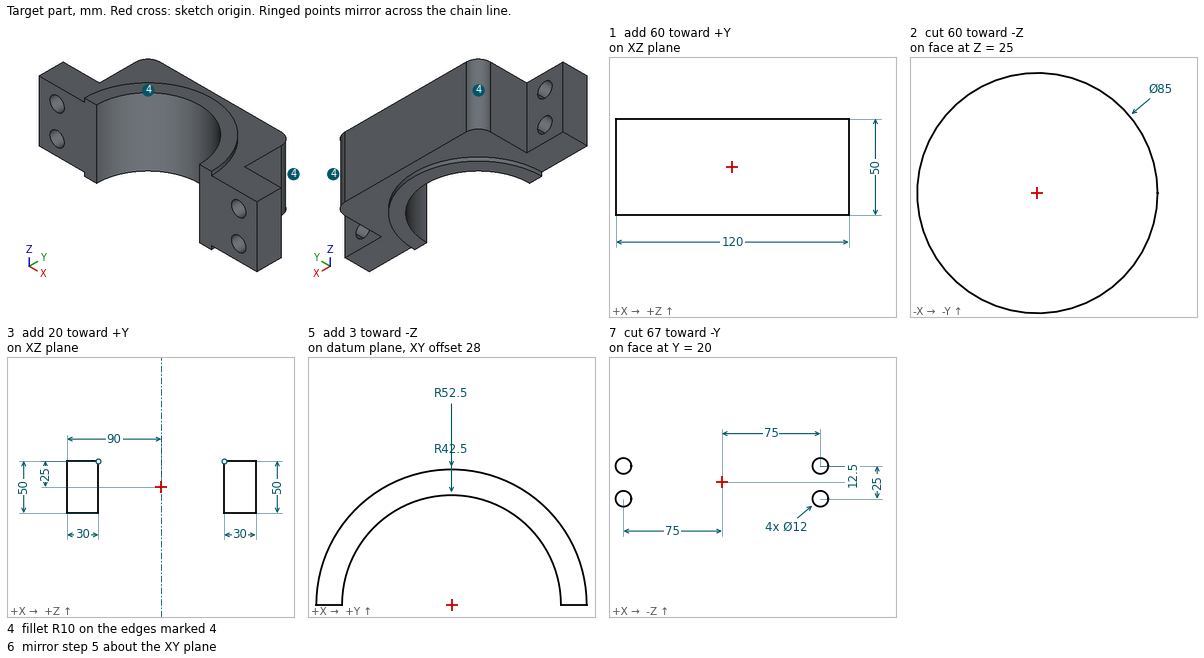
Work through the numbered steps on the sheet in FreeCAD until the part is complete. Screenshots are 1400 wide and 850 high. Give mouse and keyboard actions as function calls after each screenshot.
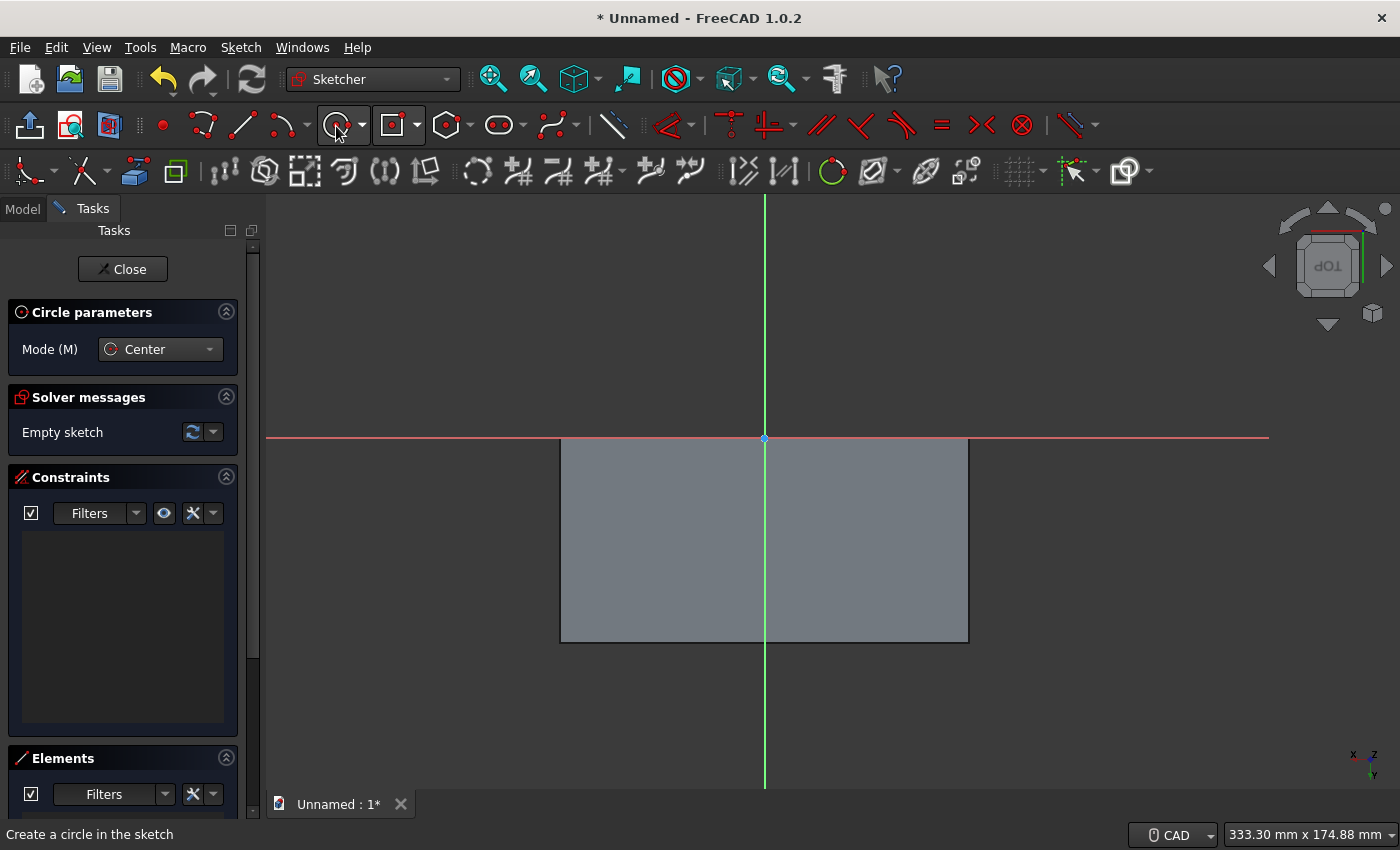
click(765, 438)
move(867, 336)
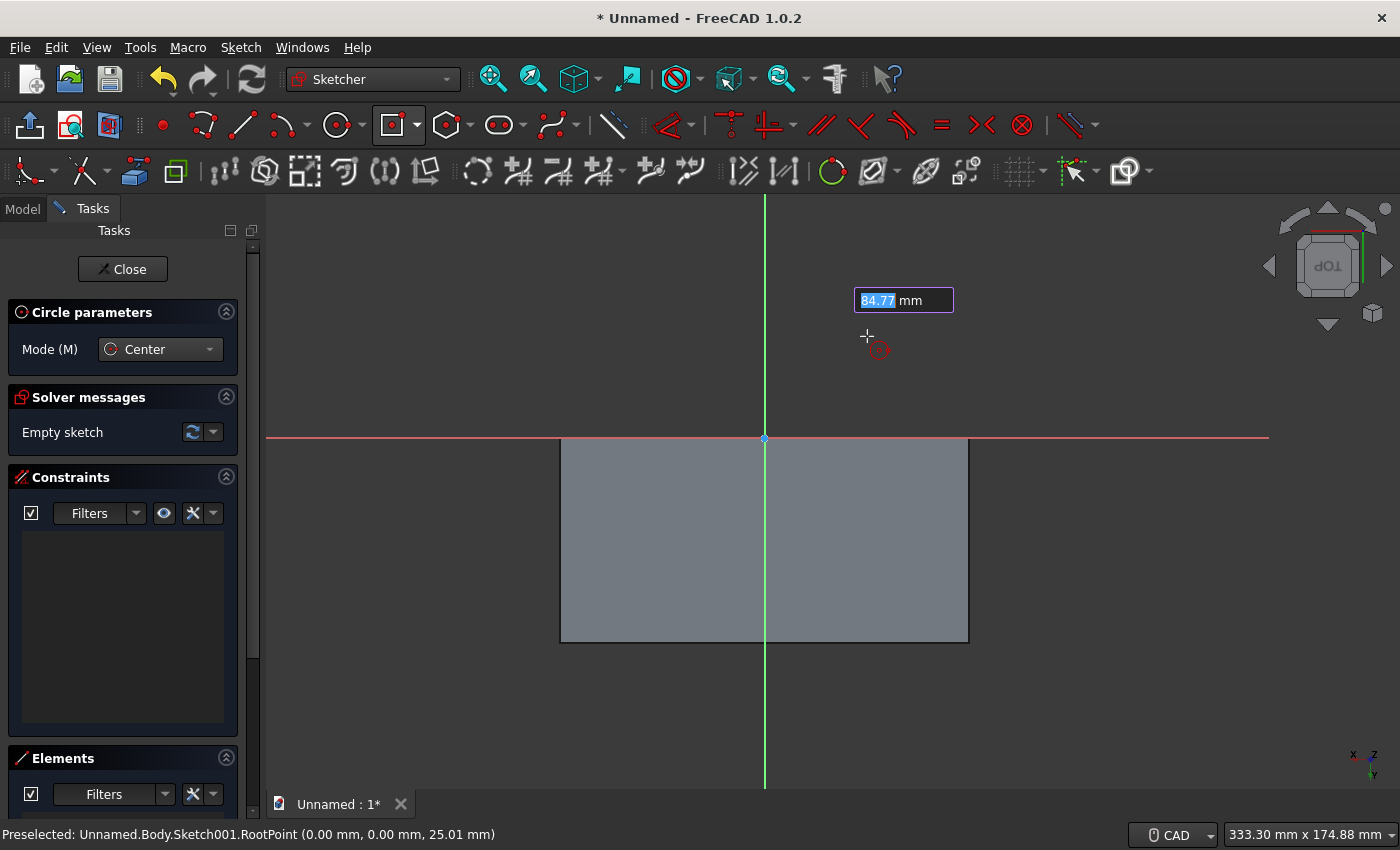
text(85)
key(Return)
key(Escape)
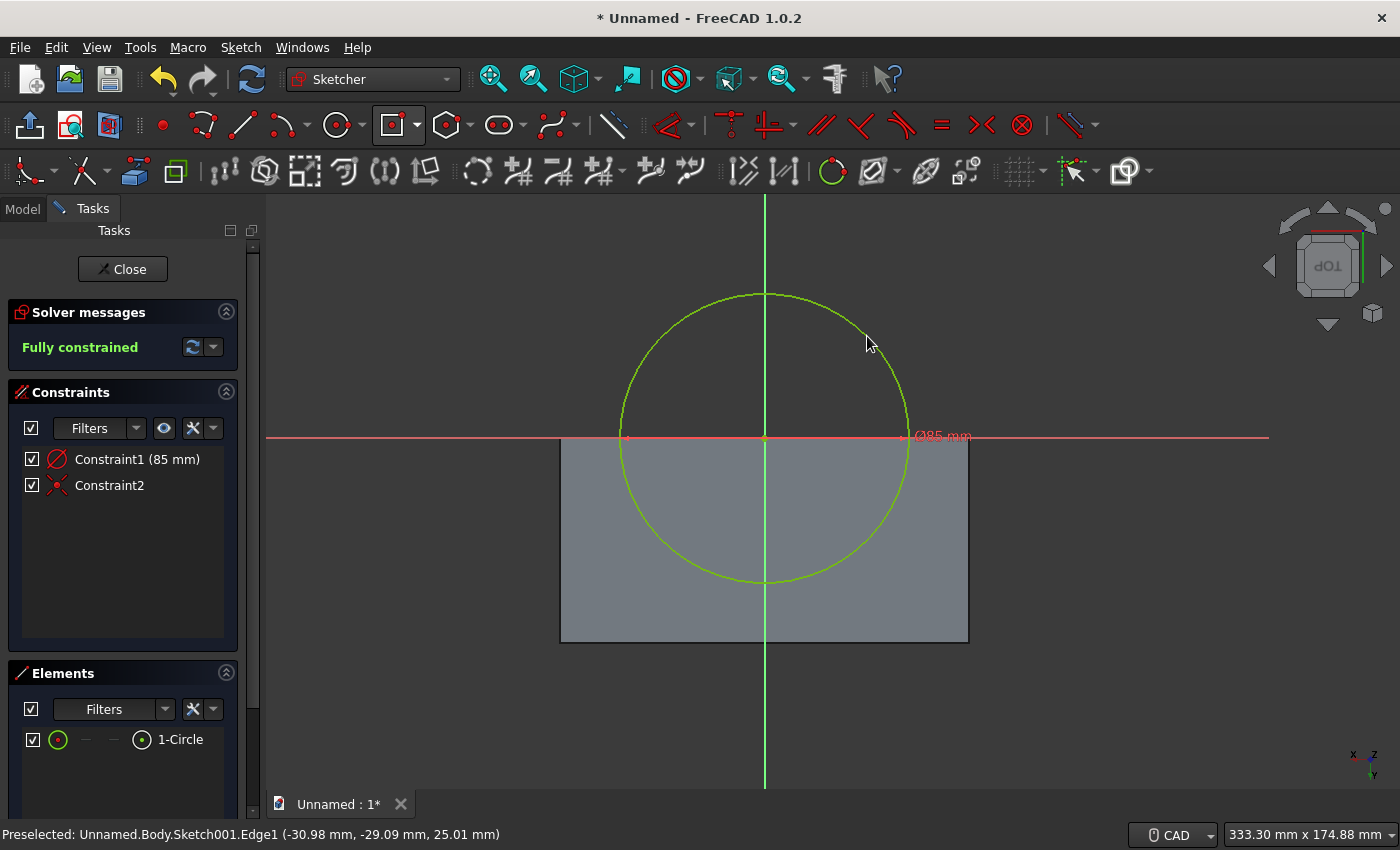
click(123, 269)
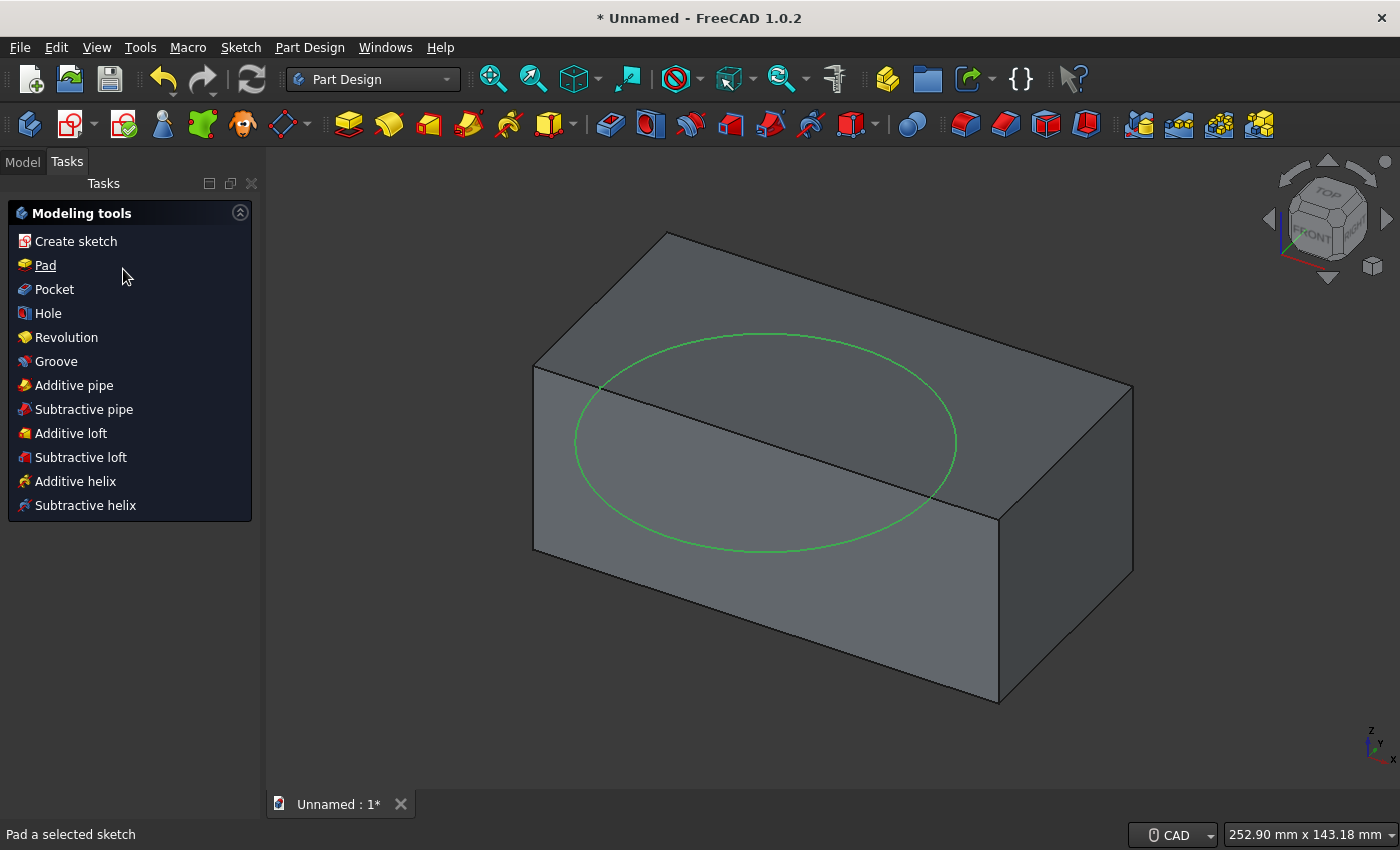
click(612, 124)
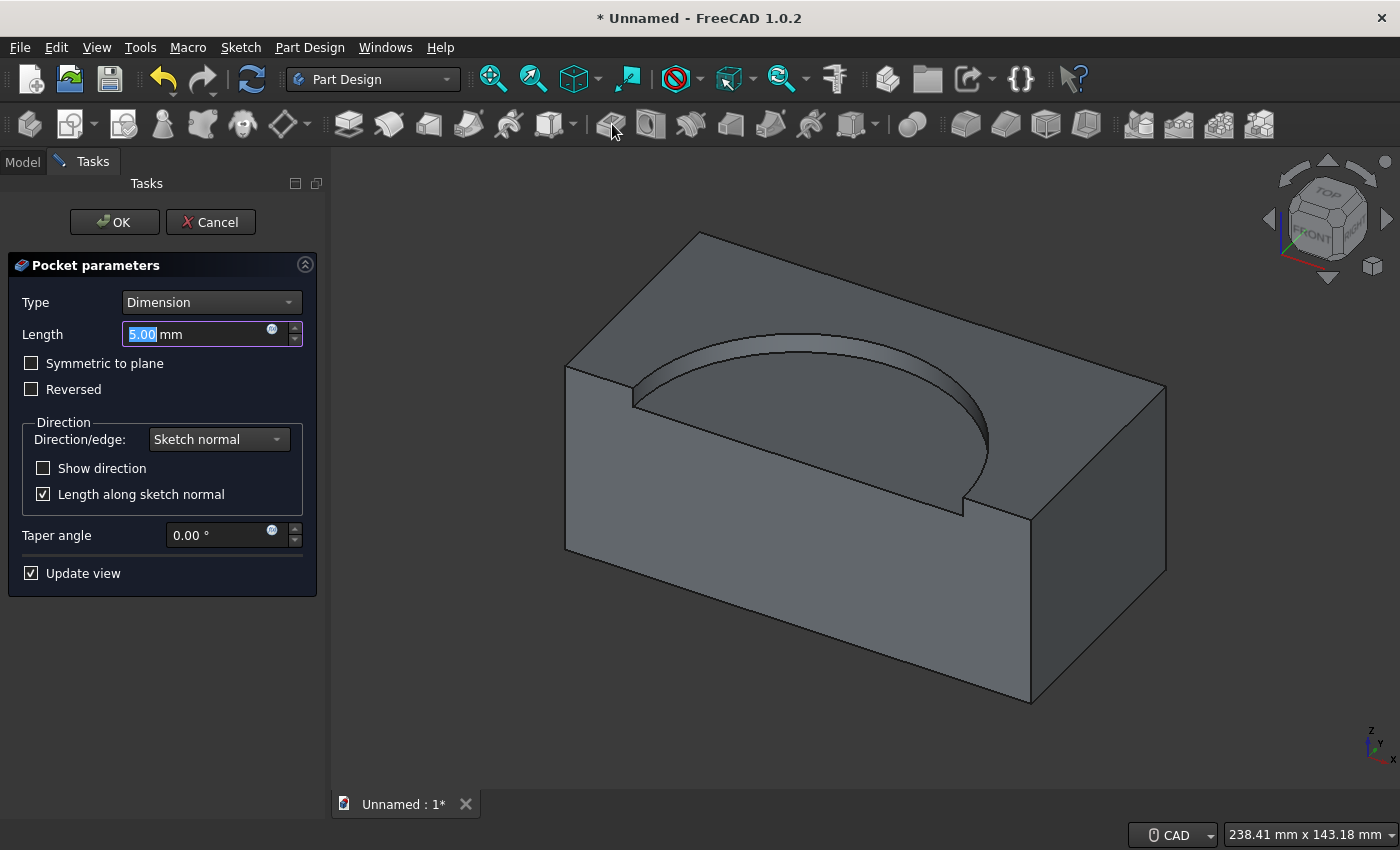
text(60)
key(Tab)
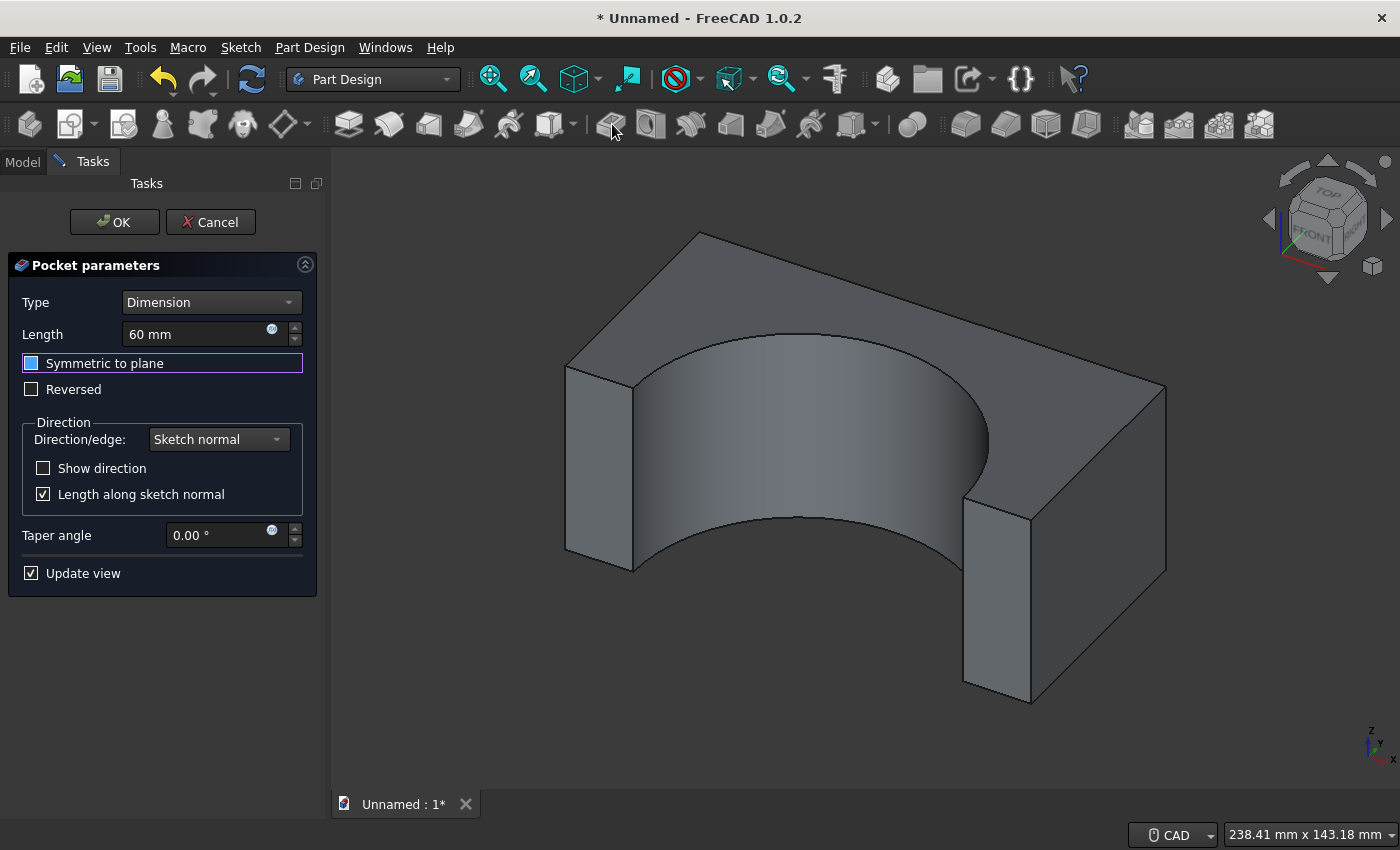
click(115, 222)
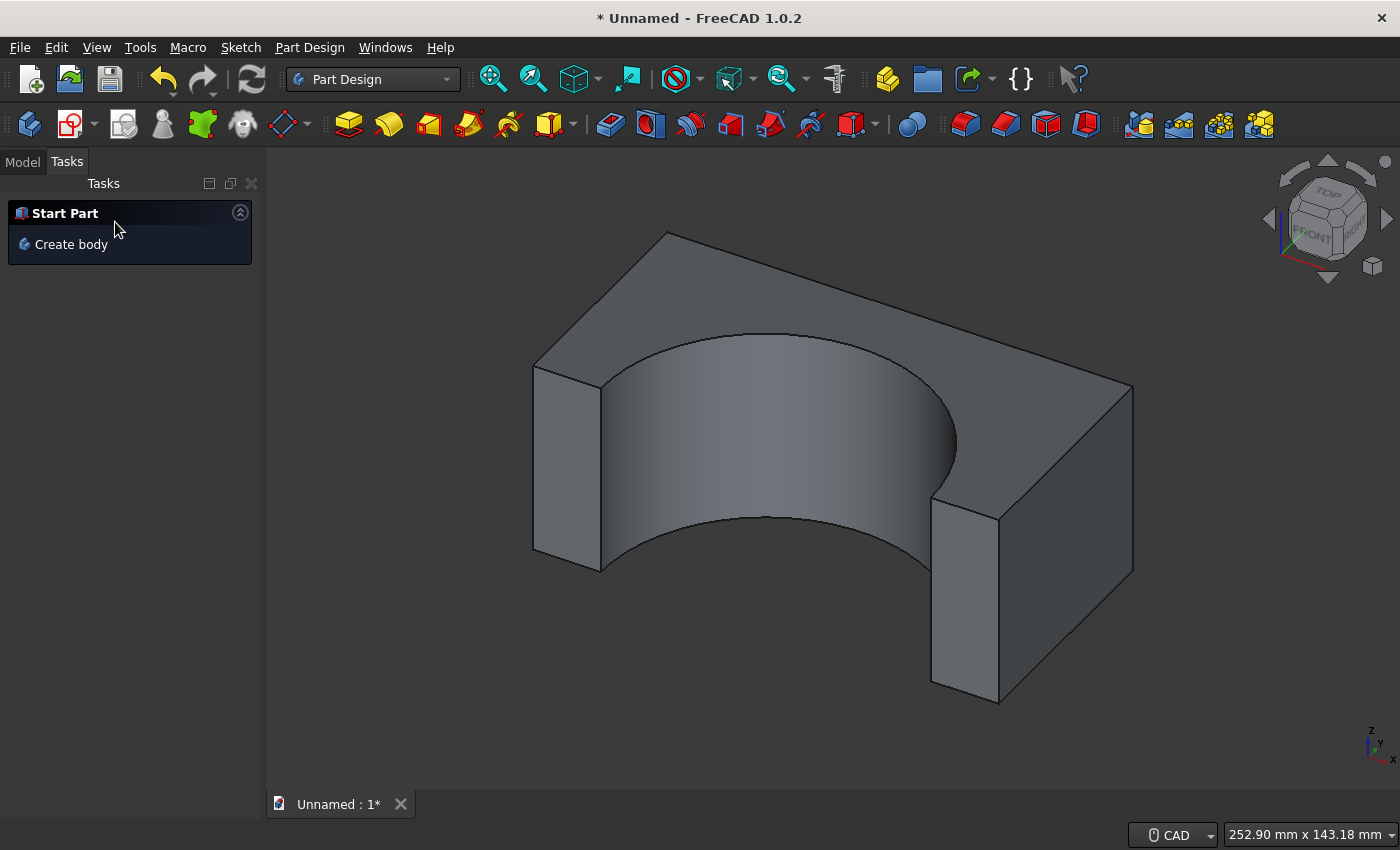
click(70, 124)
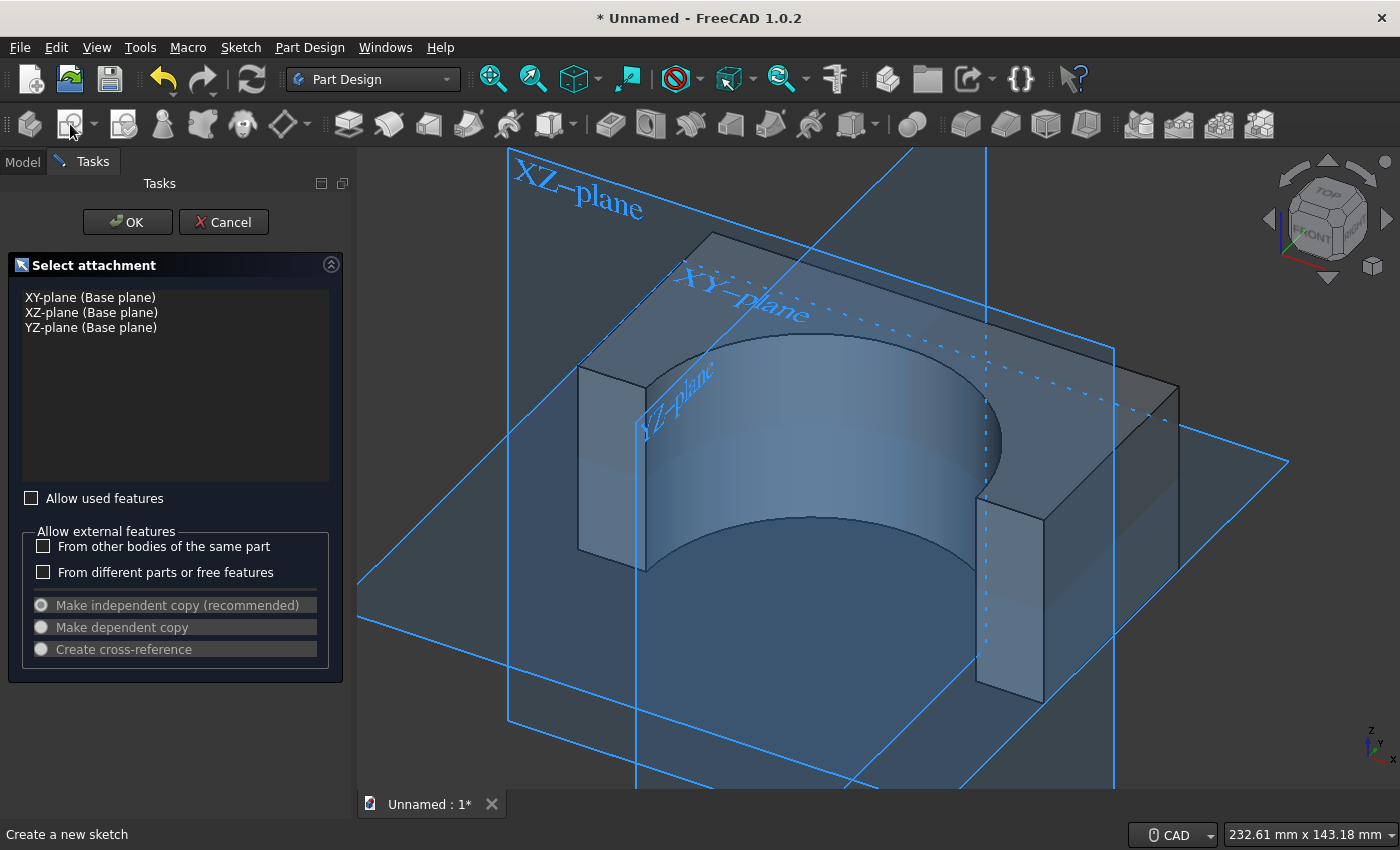
click(82, 312)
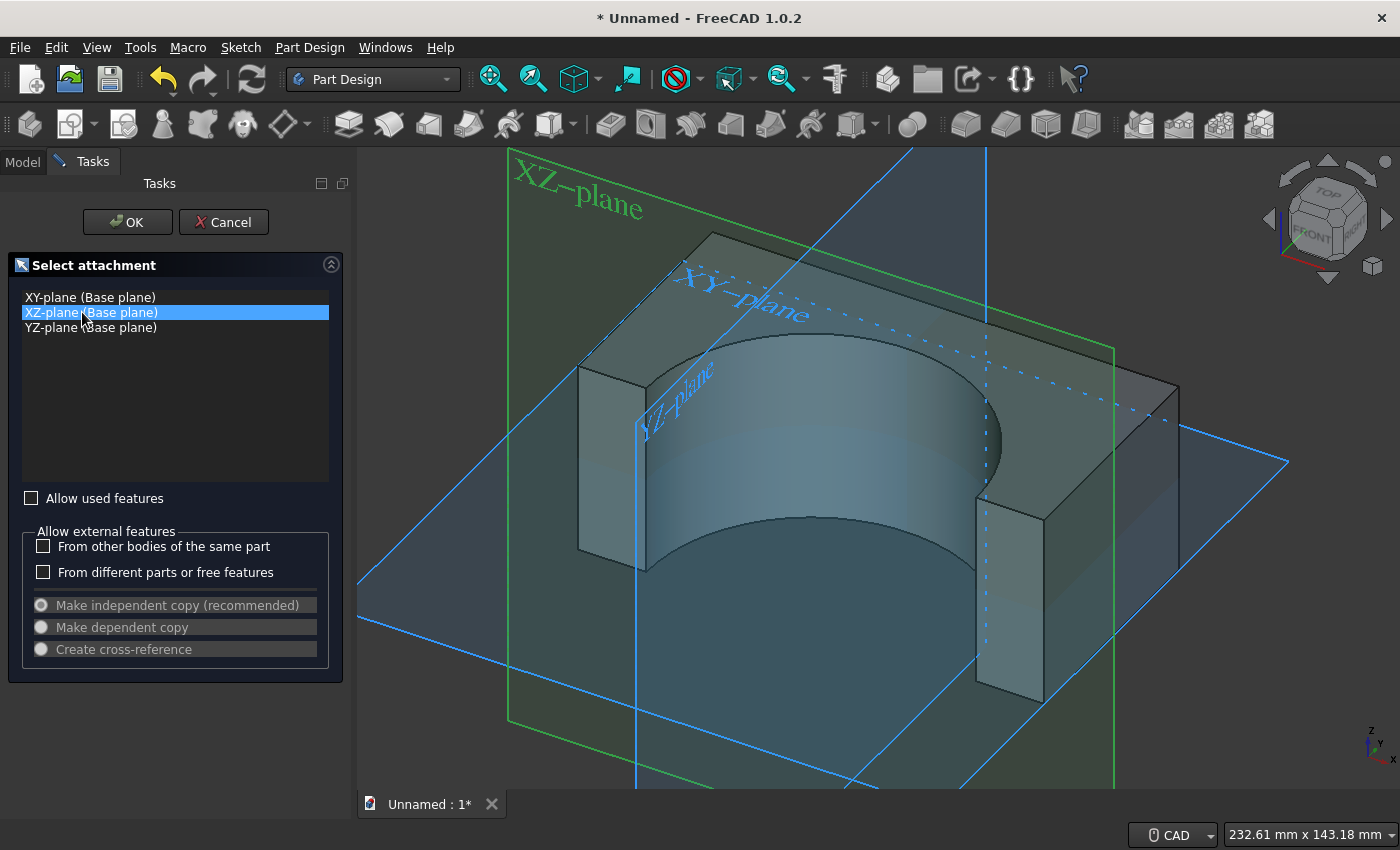
click(128, 222)